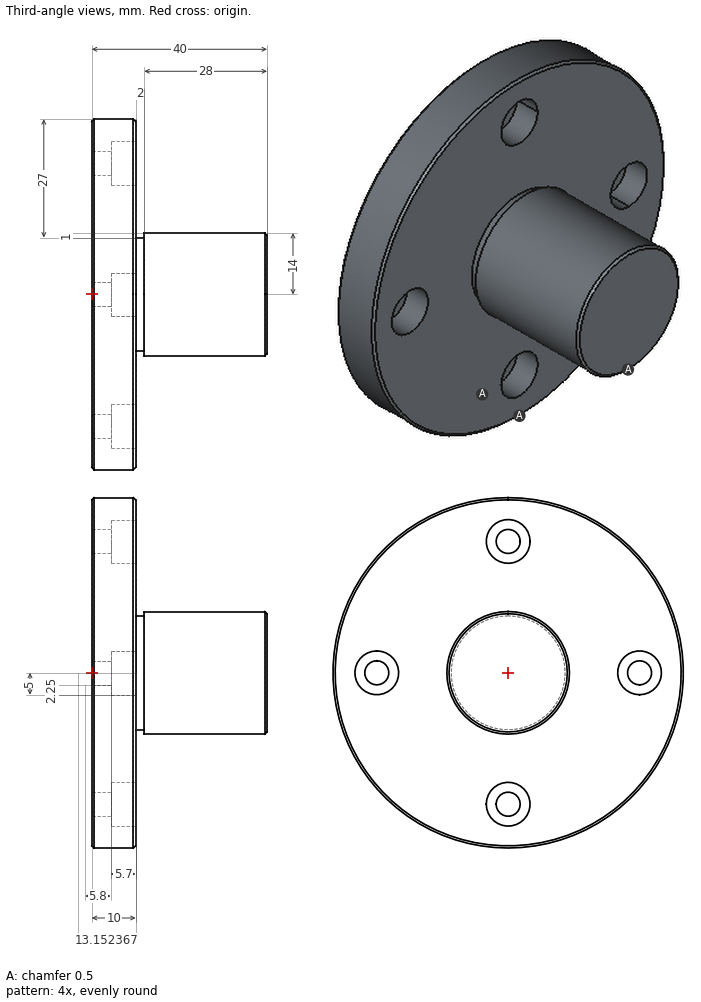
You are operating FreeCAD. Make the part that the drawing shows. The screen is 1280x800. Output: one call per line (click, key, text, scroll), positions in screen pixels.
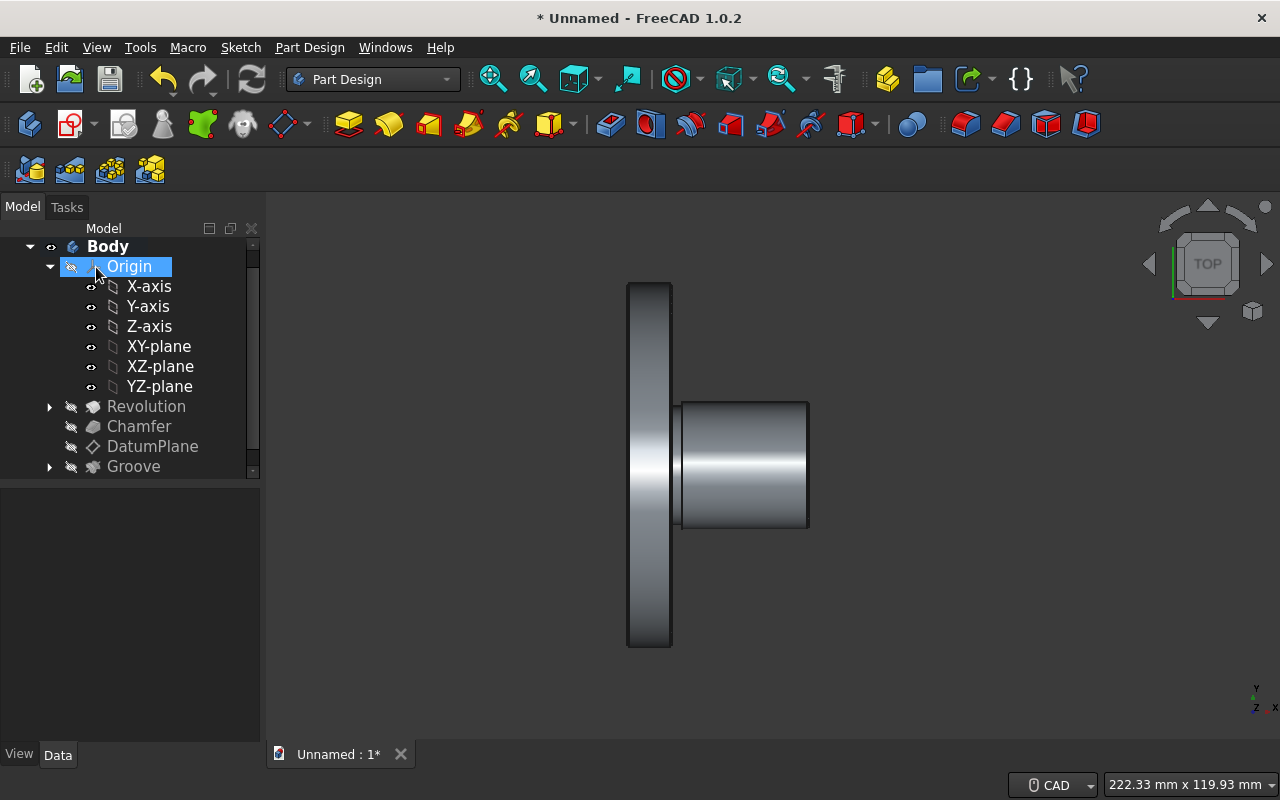
key(0)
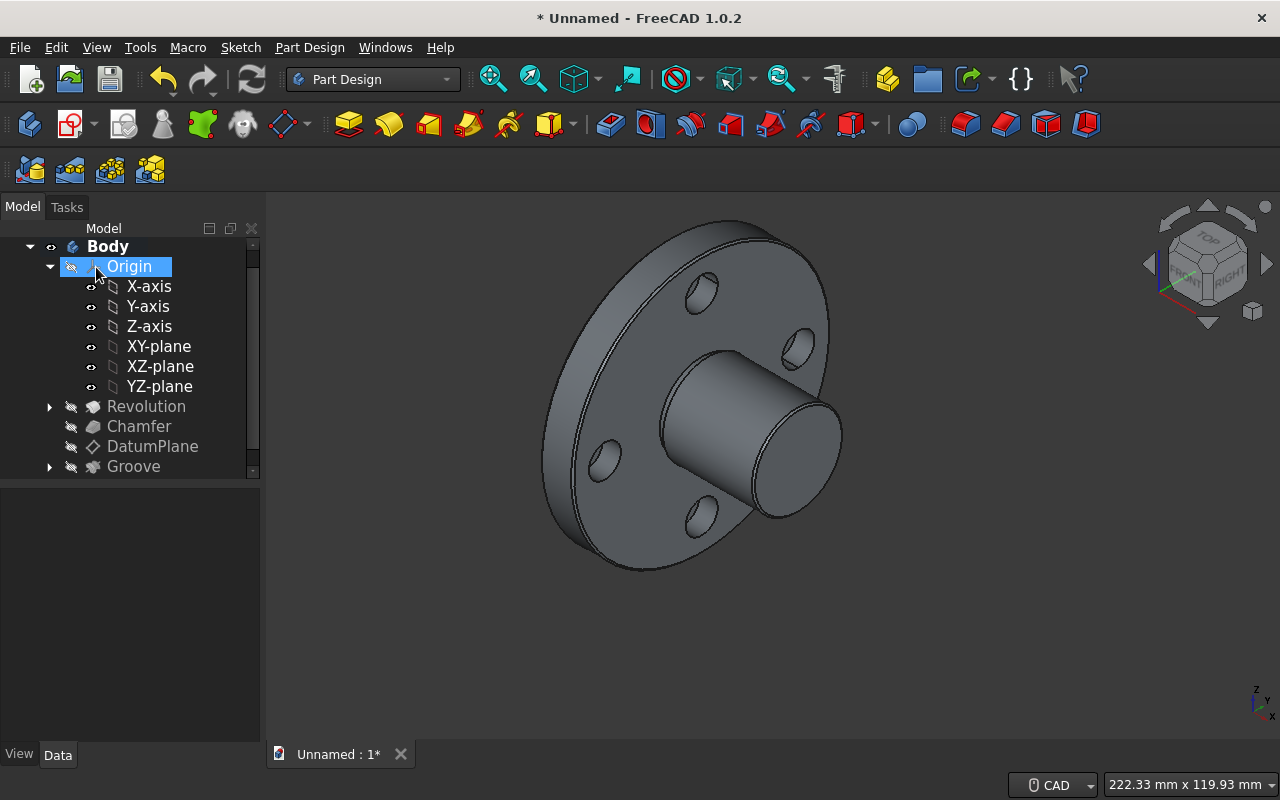
click(494, 80)